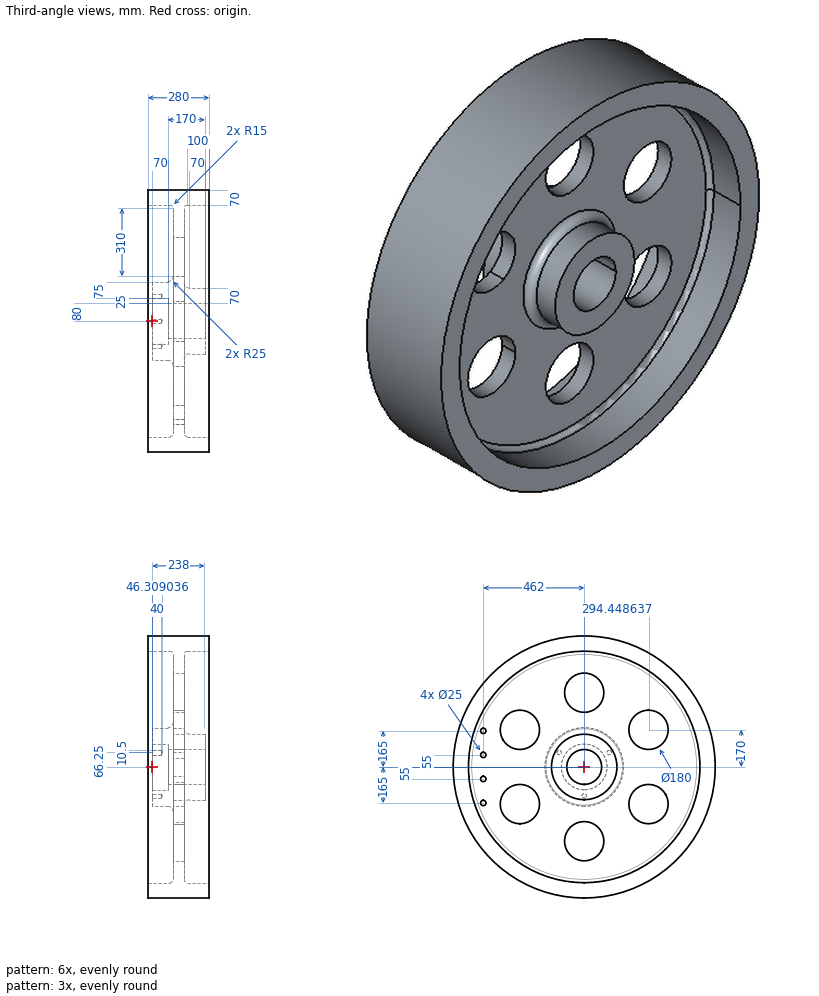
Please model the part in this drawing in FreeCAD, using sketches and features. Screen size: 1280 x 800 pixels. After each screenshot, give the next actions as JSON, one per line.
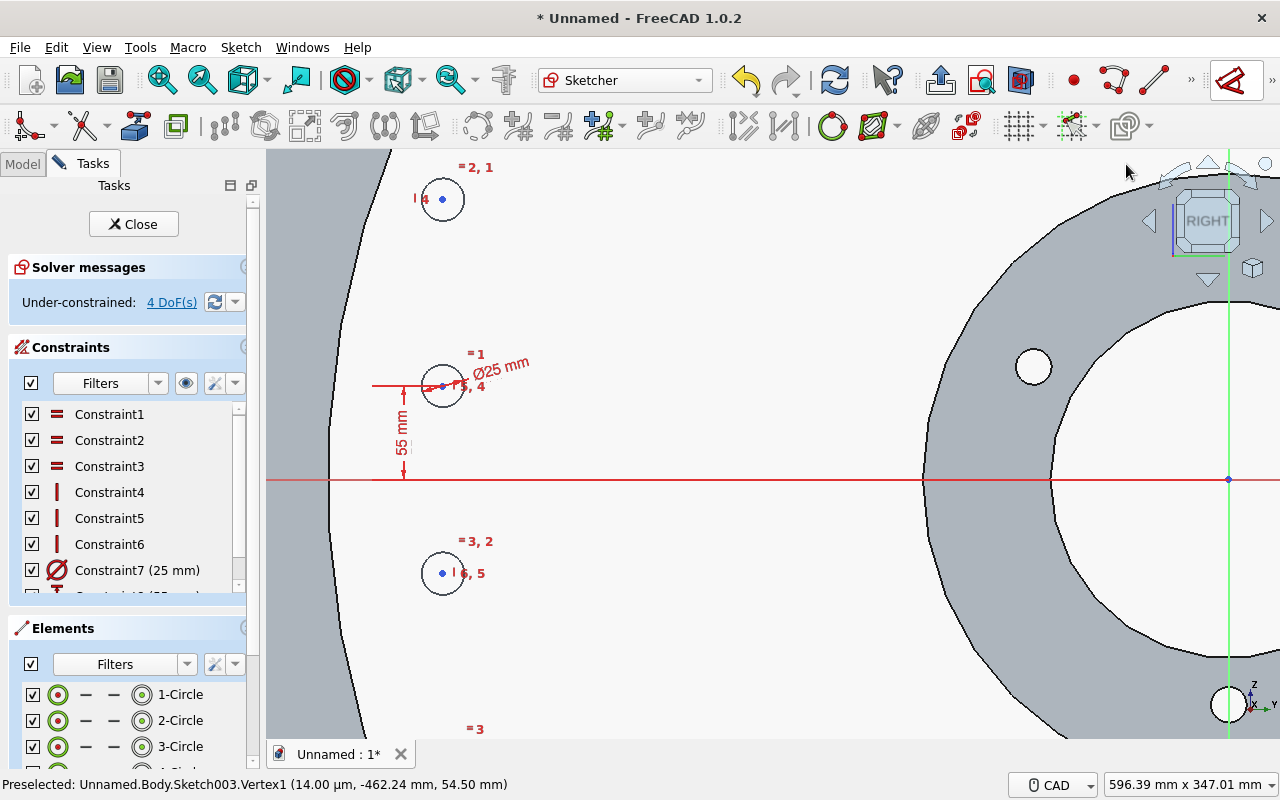
{"action": "left_click", "coordinate": [443, 574]}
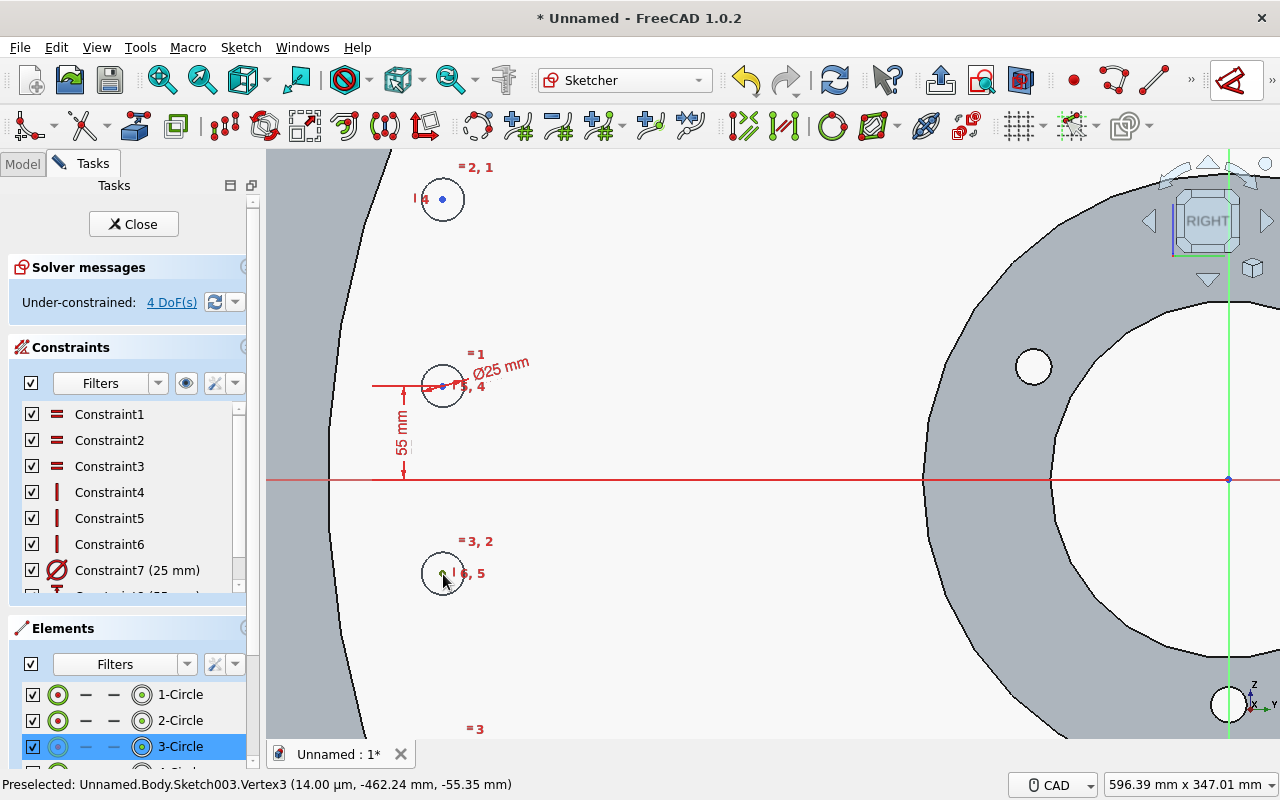
{"action": "key", "text": "i"}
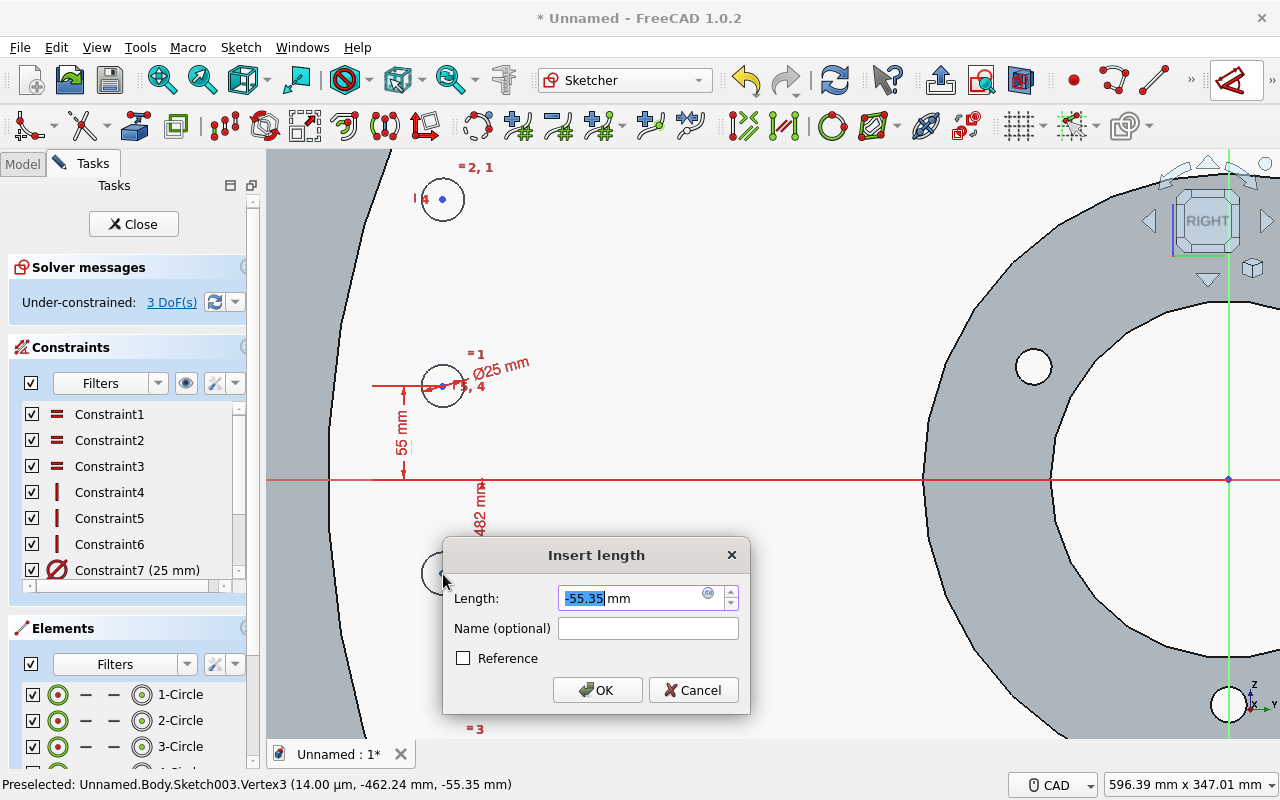
{"action": "type", "text": "-55"}
{"action": "key", "text": "Return"}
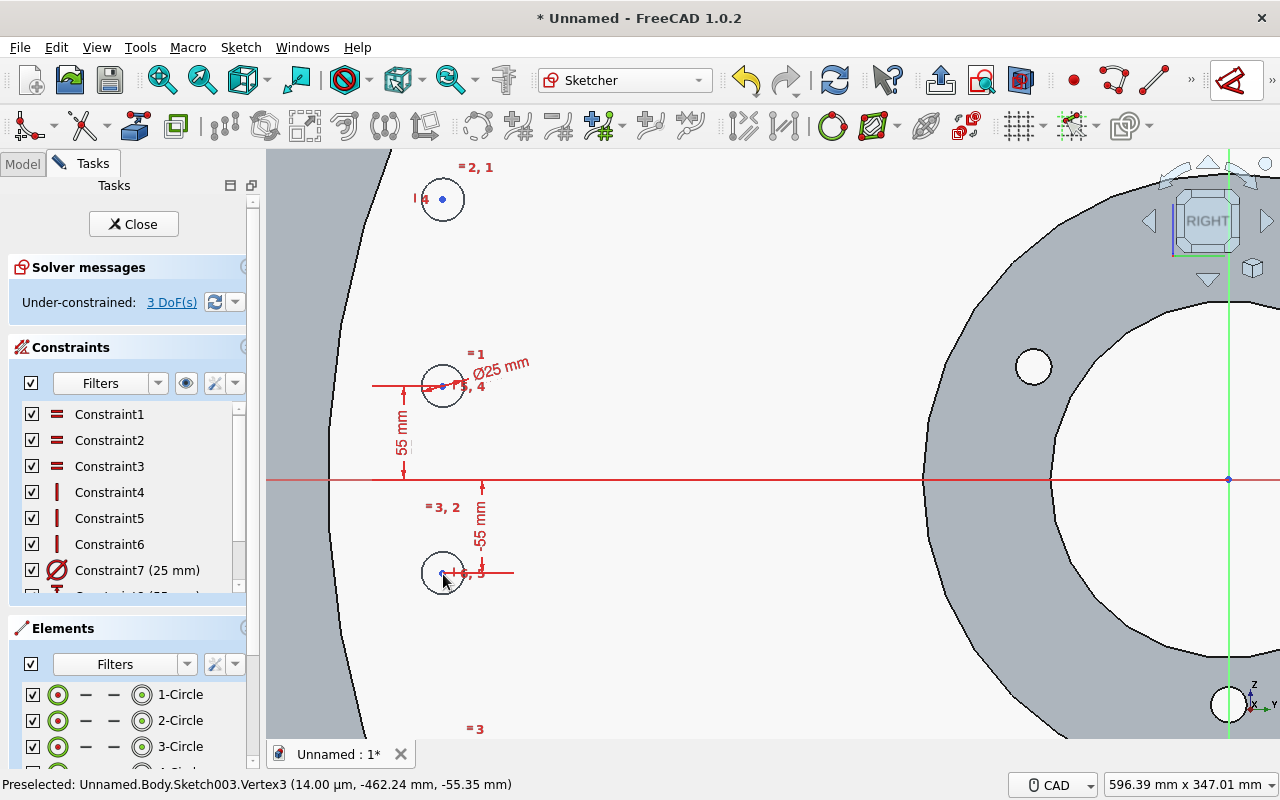
{"action": "left_click", "coordinate": [443, 386]}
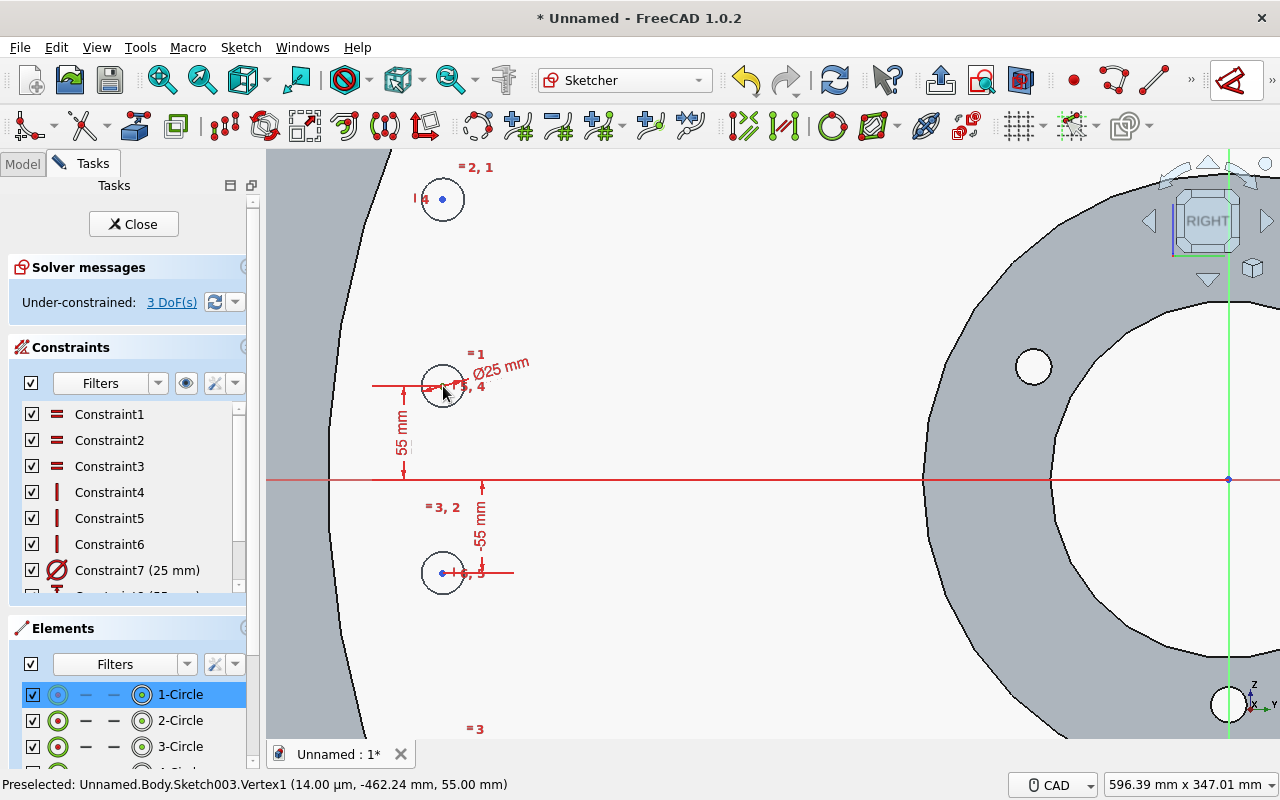
{"action": "left_click", "coordinate": [1258, 80]}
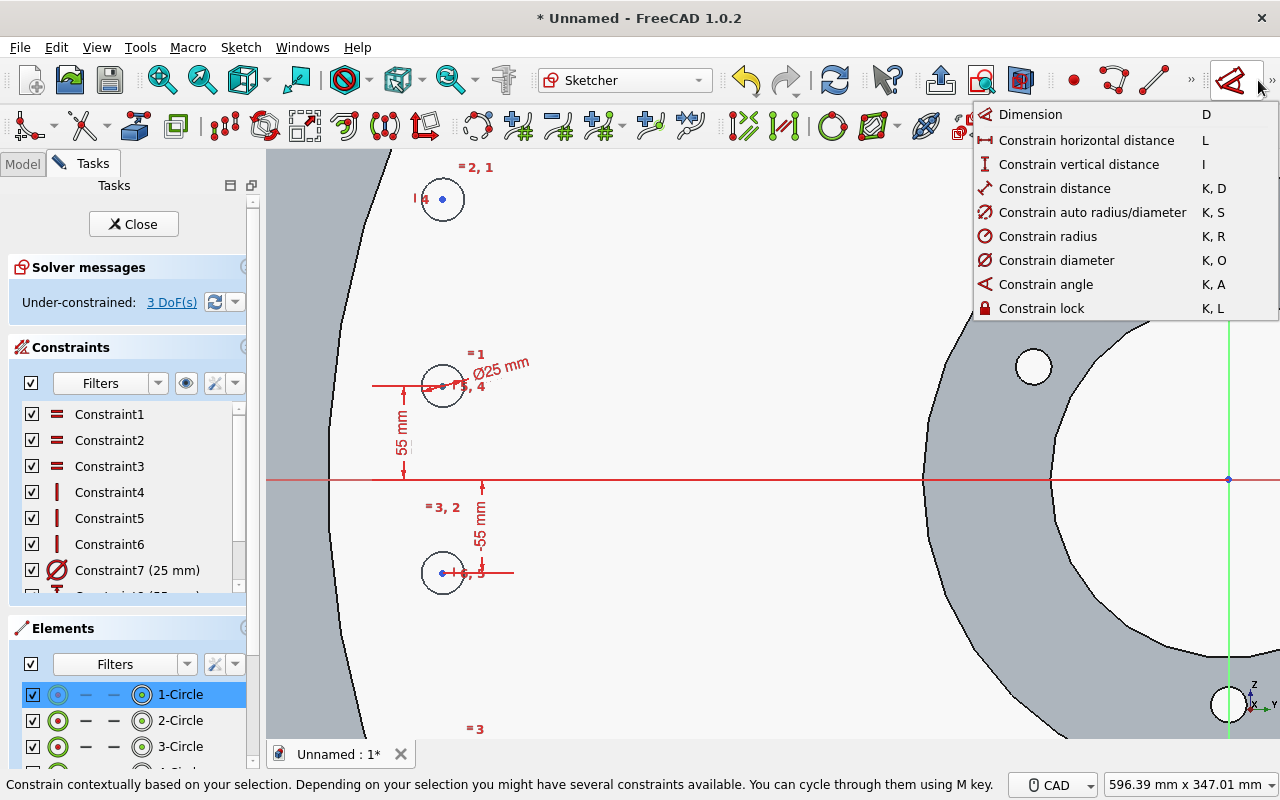
{"action": "left_click", "coordinate": [1126, 140]}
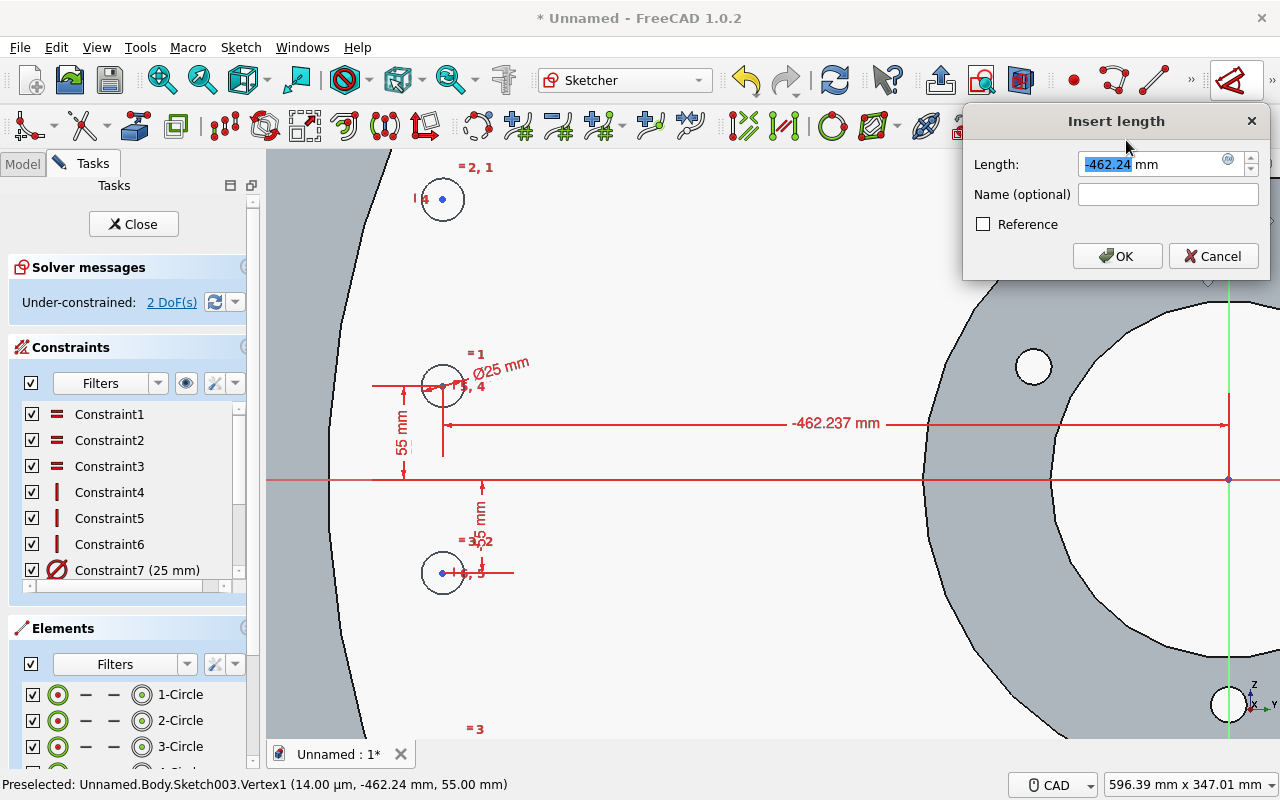
{"action": "type", "text": "-462"}
{"action": "key", "text": "Return"}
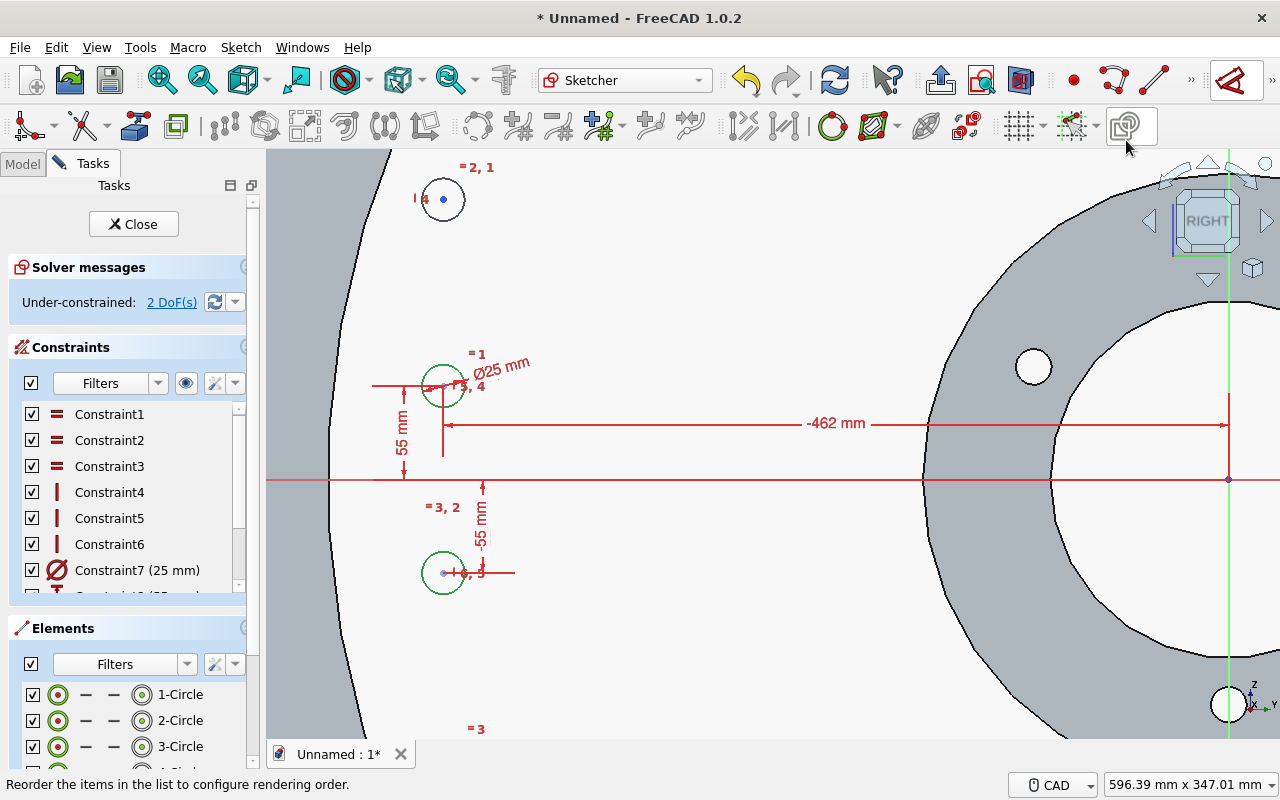
{"action": "left_click", "coordinate": [443, 200]}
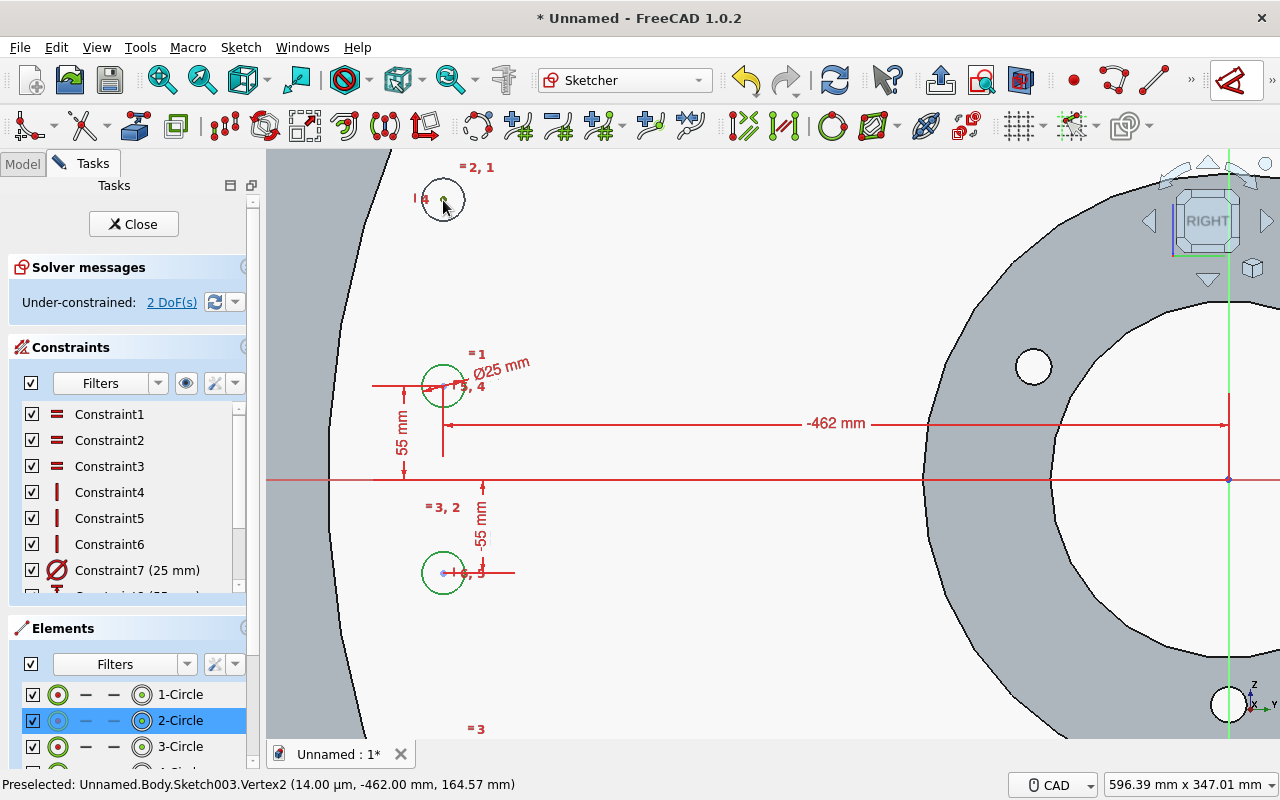
{"action": "key", "text": "i"}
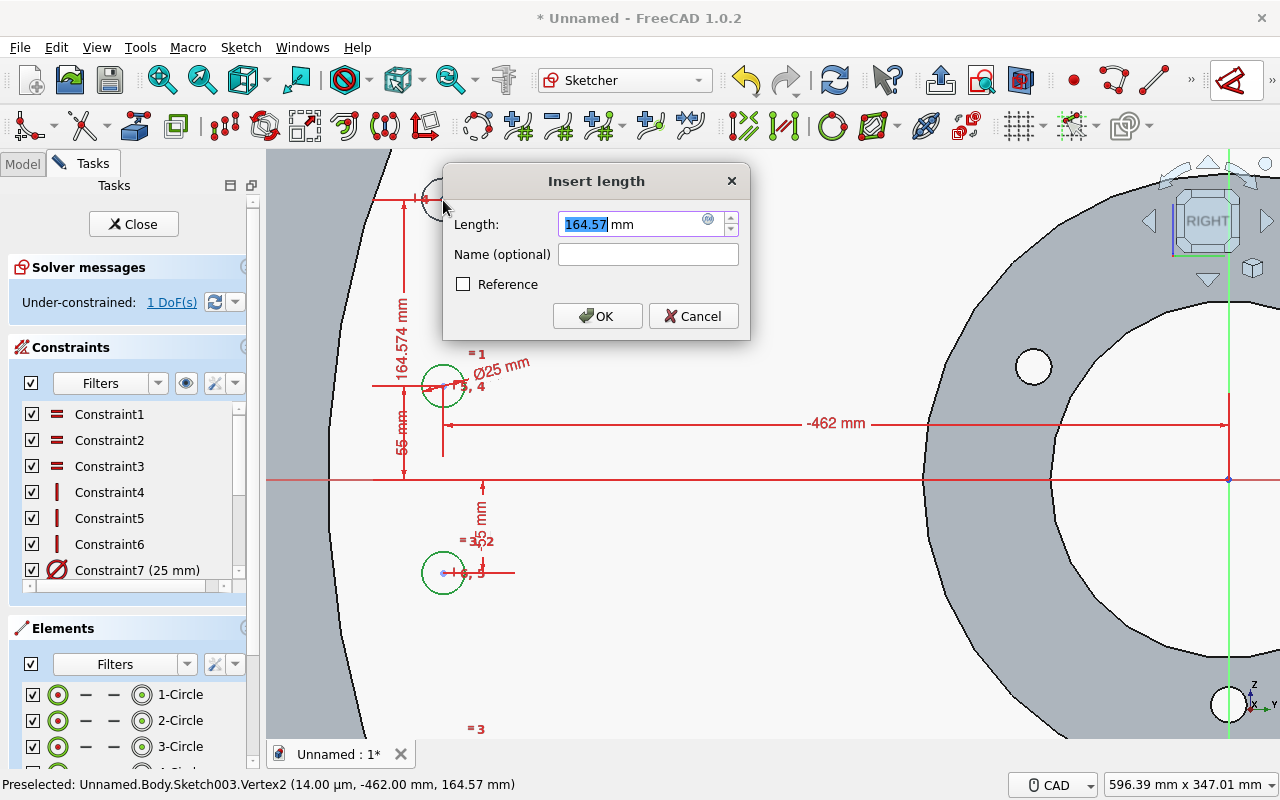
{"action": "type", "text": "165"}
{"action": "key", "text": "Return"}